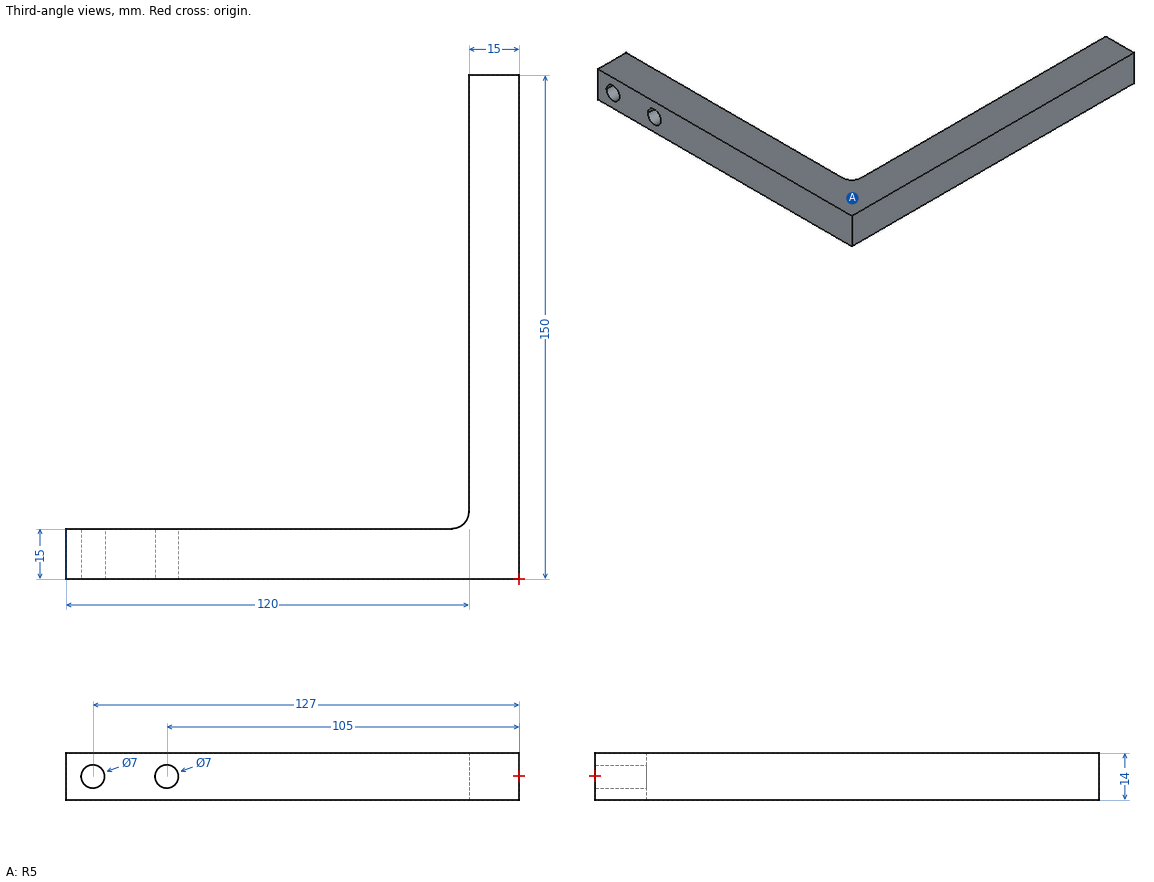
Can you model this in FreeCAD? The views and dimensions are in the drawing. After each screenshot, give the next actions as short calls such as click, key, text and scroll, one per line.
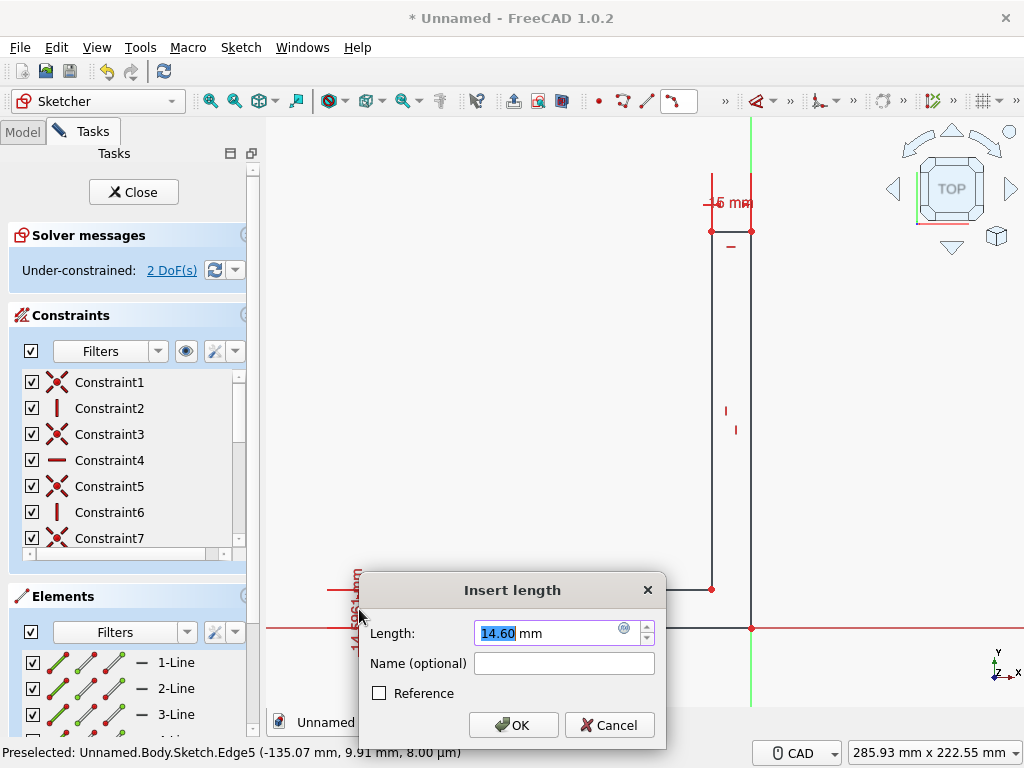
text(15)
key(Return)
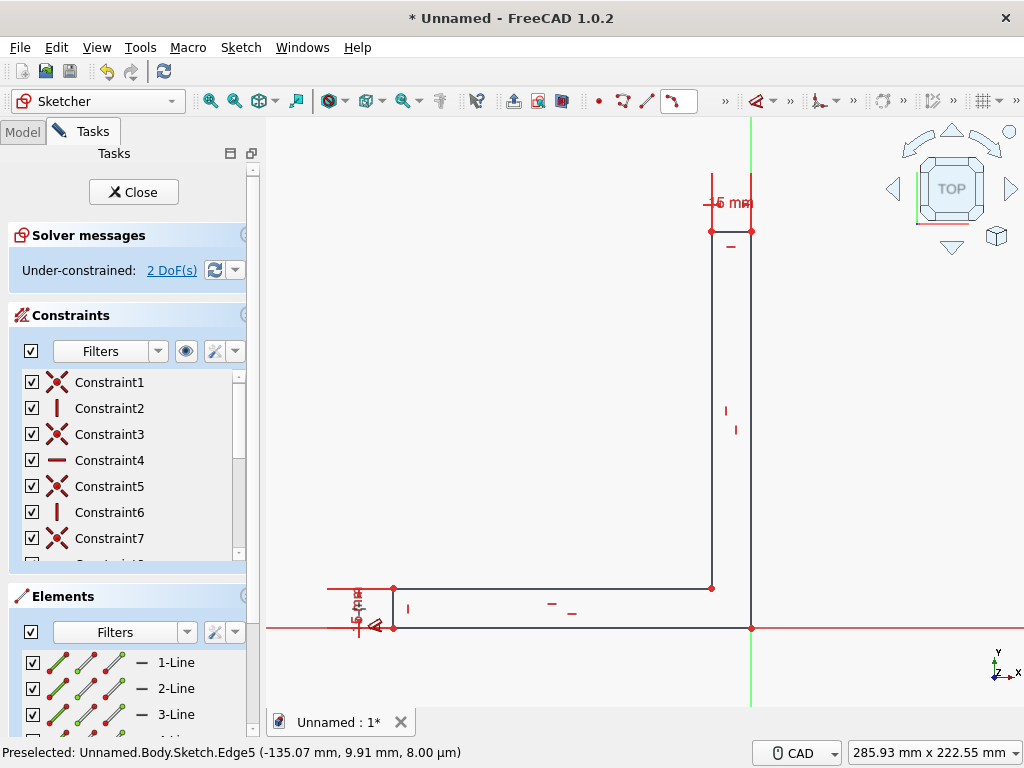
click(751, 509)
click(785, 430)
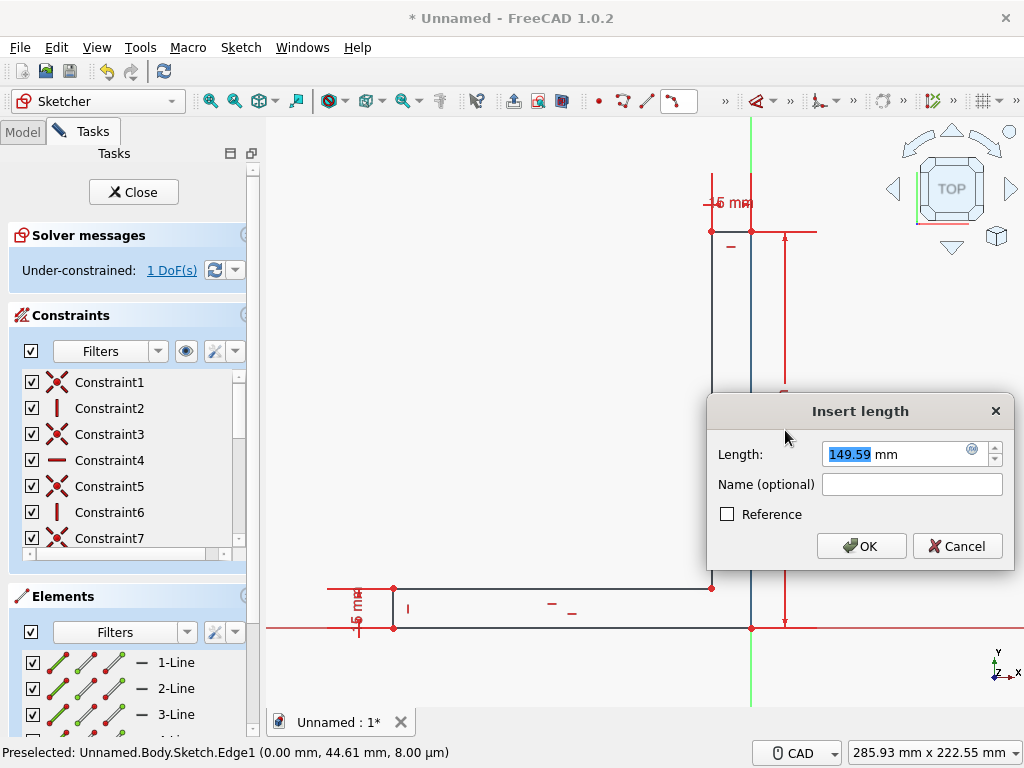
text(150)
key(Return)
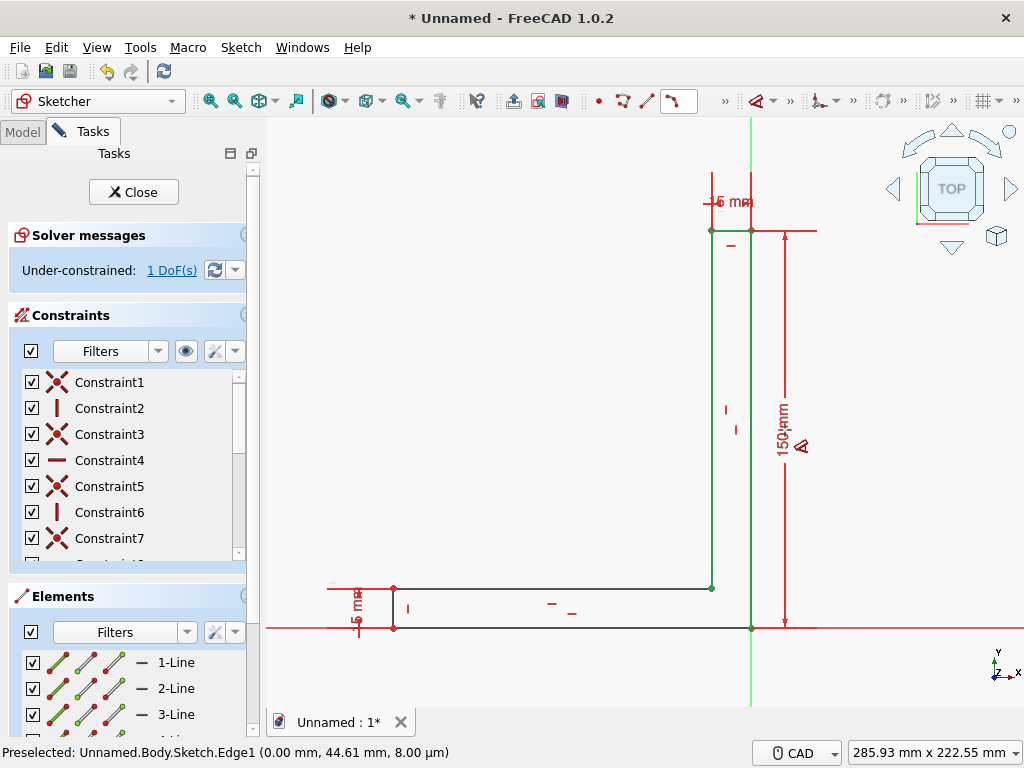
click(616, 589)
click(552, 555)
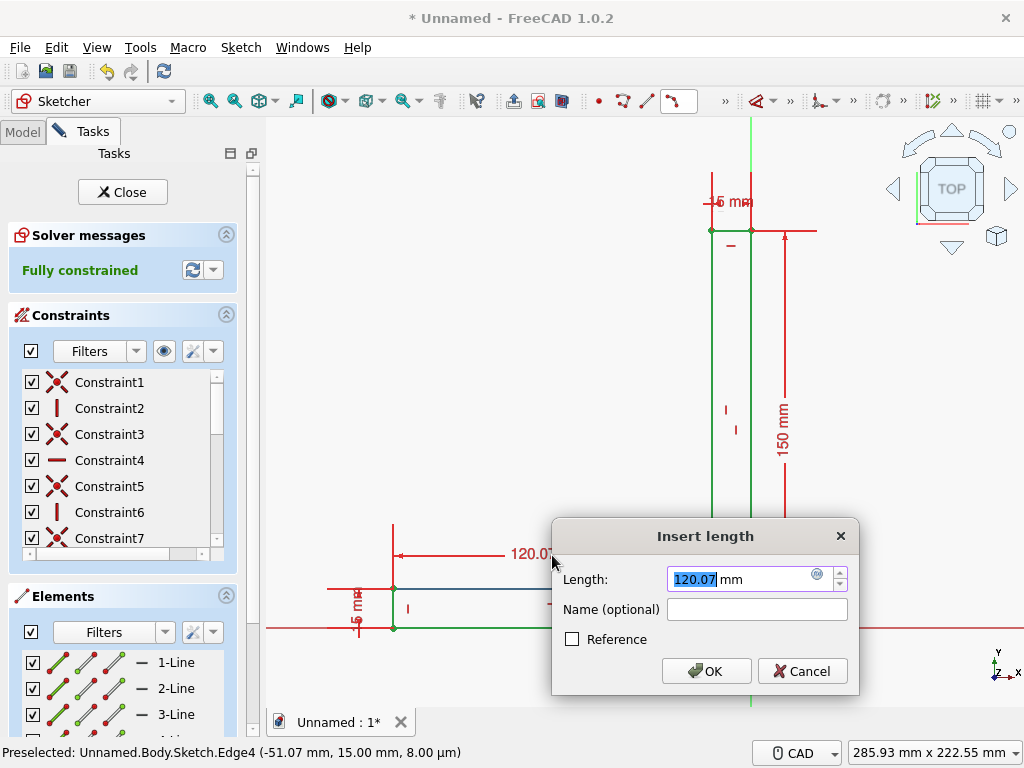
text(120)
key(Return)
key(Escape)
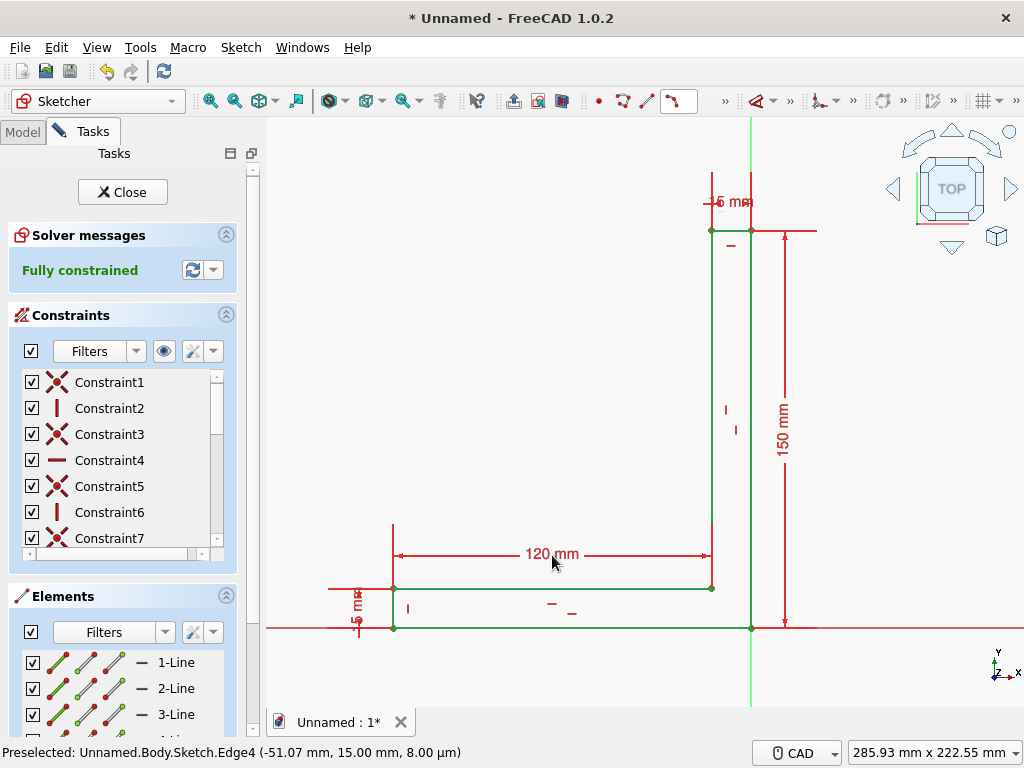
click(123, 192)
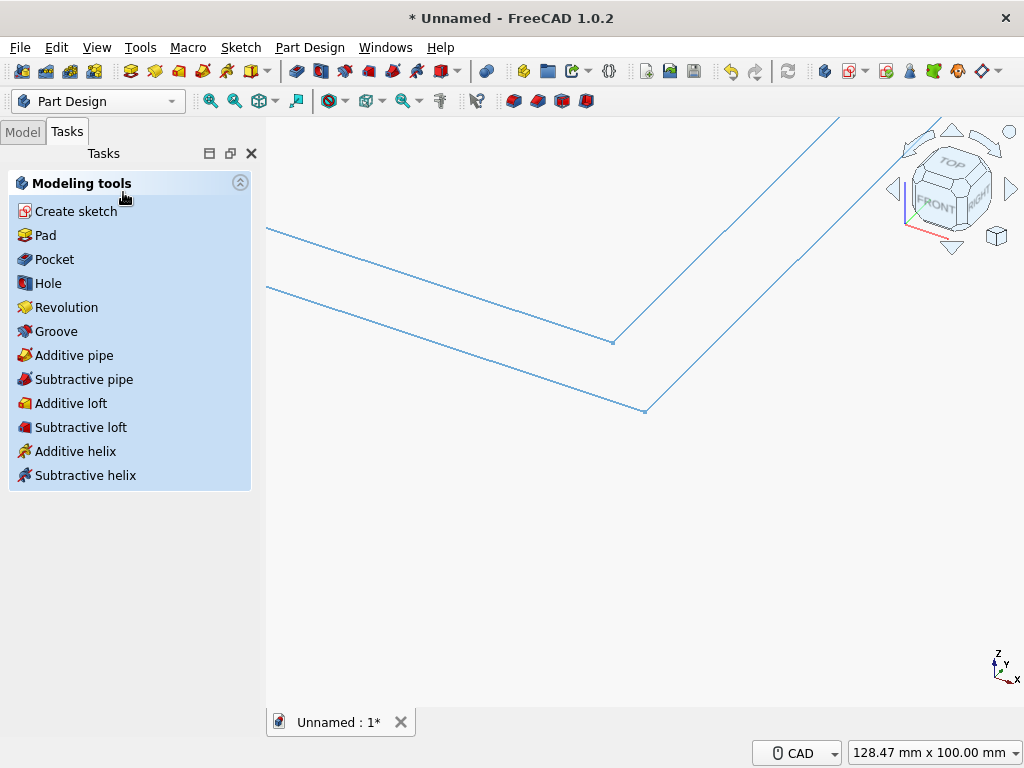
click(132, 72)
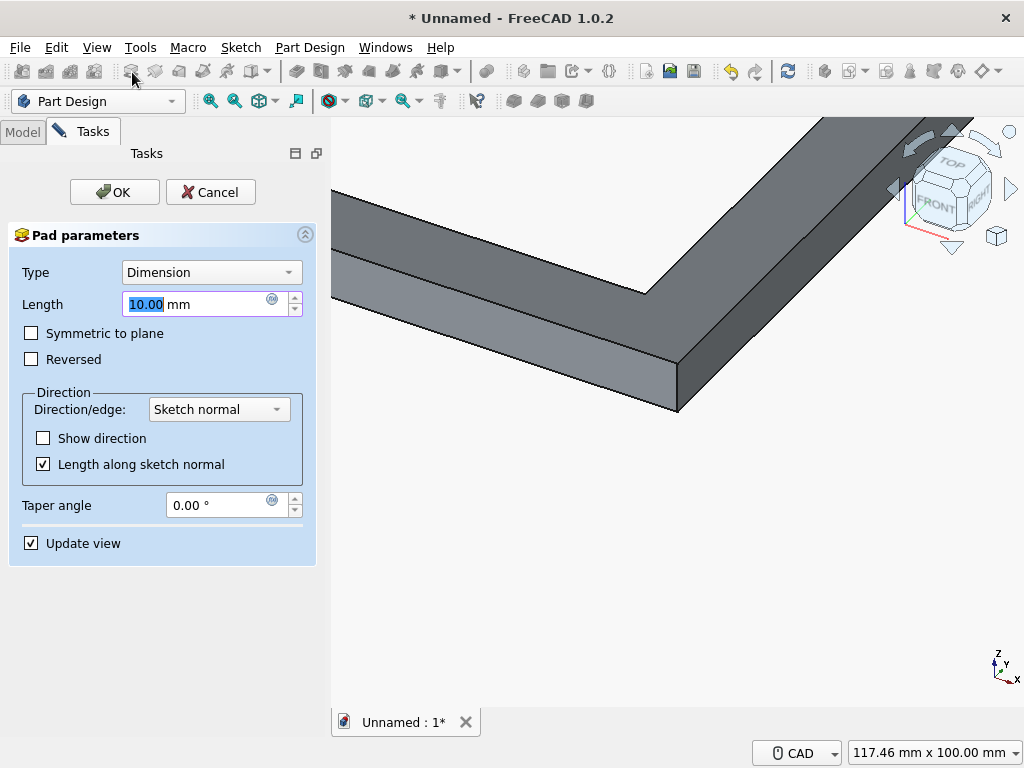
text(14)
key(Tab)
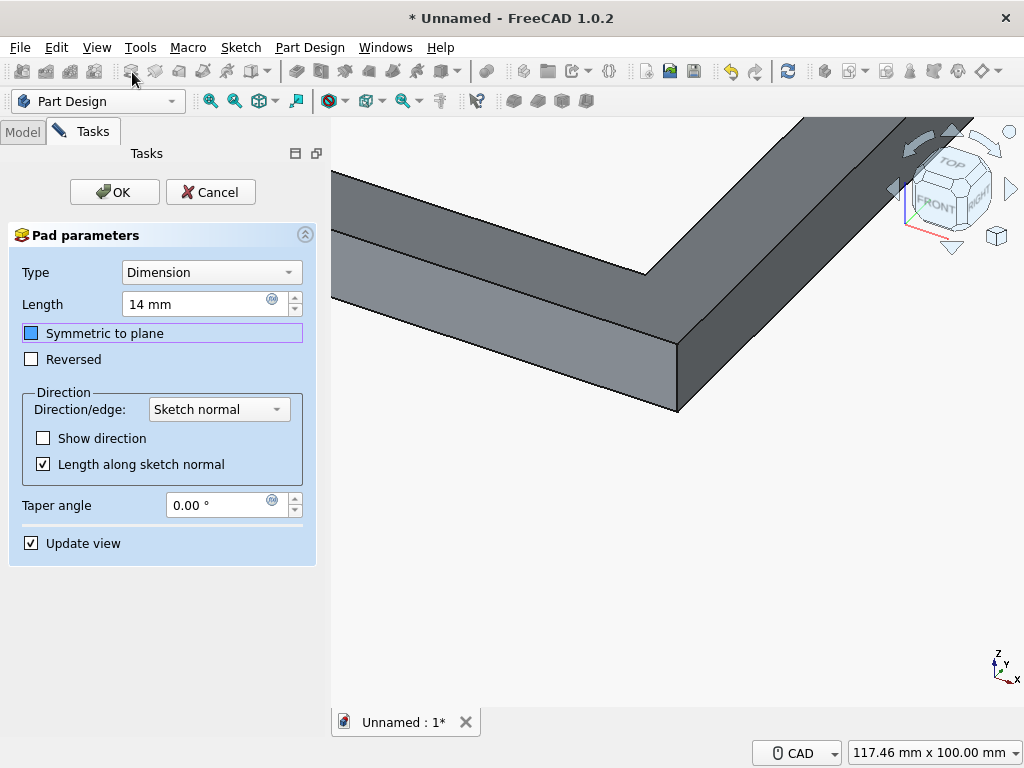
click(30, 333)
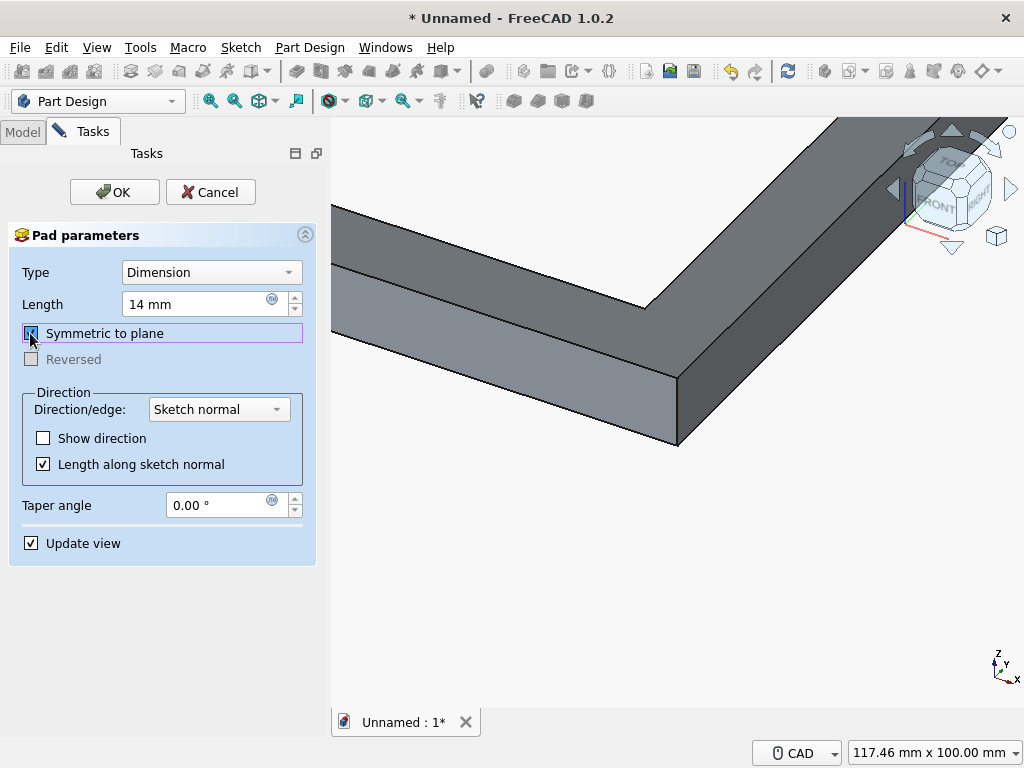
click(115, 192)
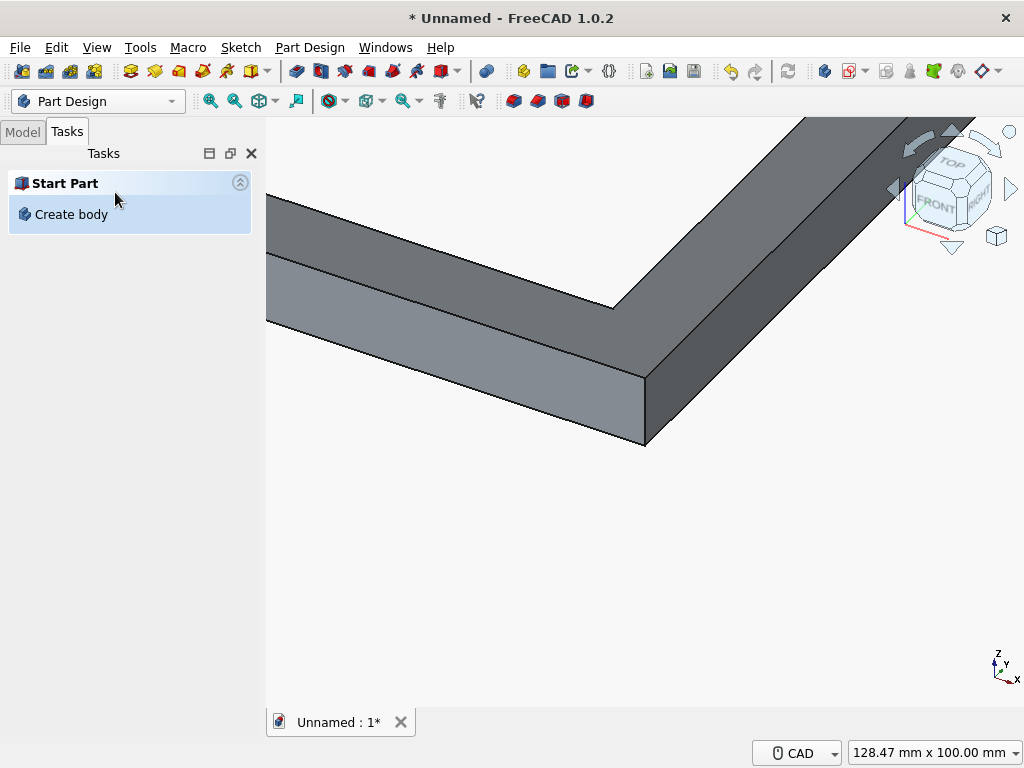
click(212, 102)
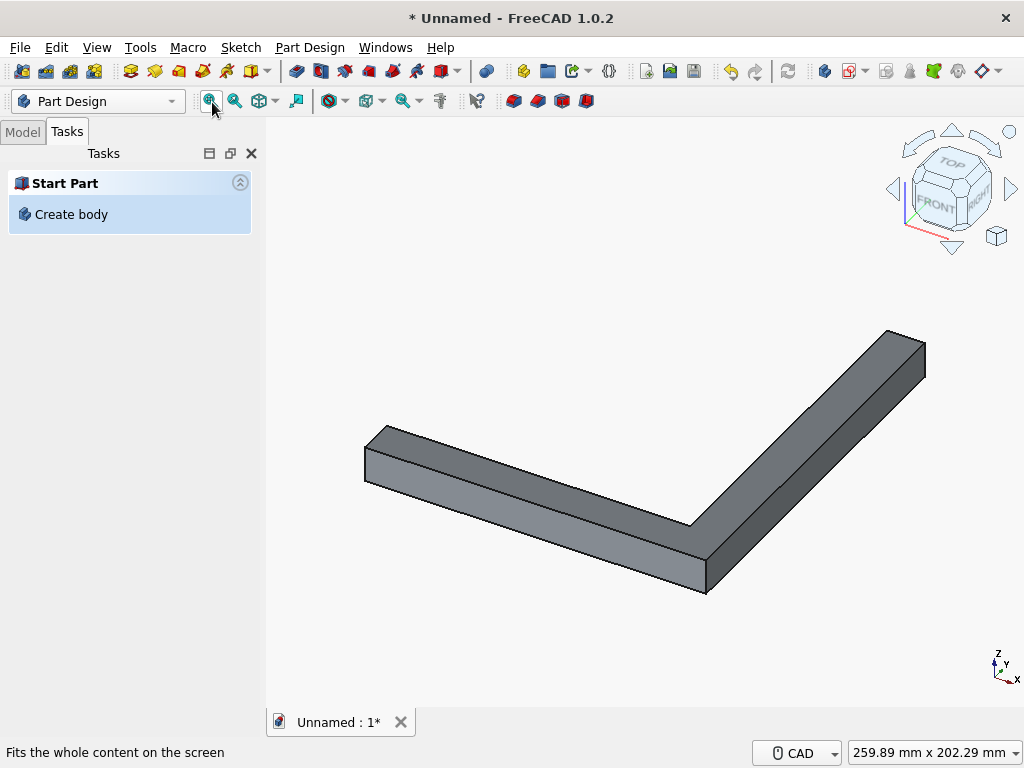
key(0)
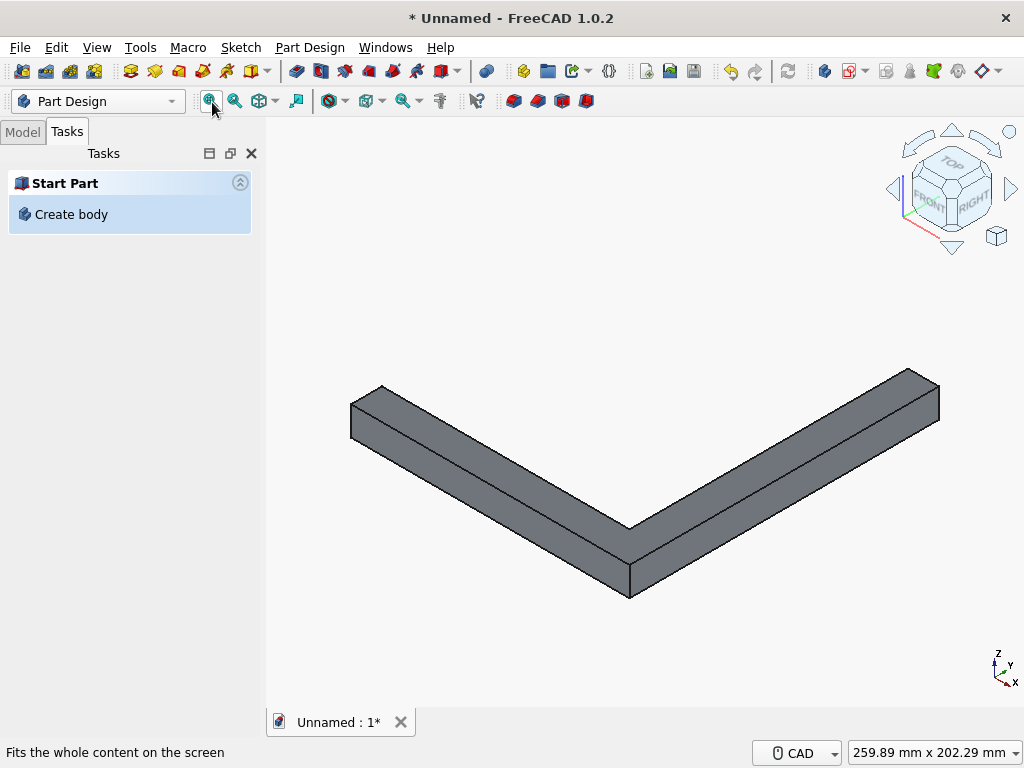
key(2)